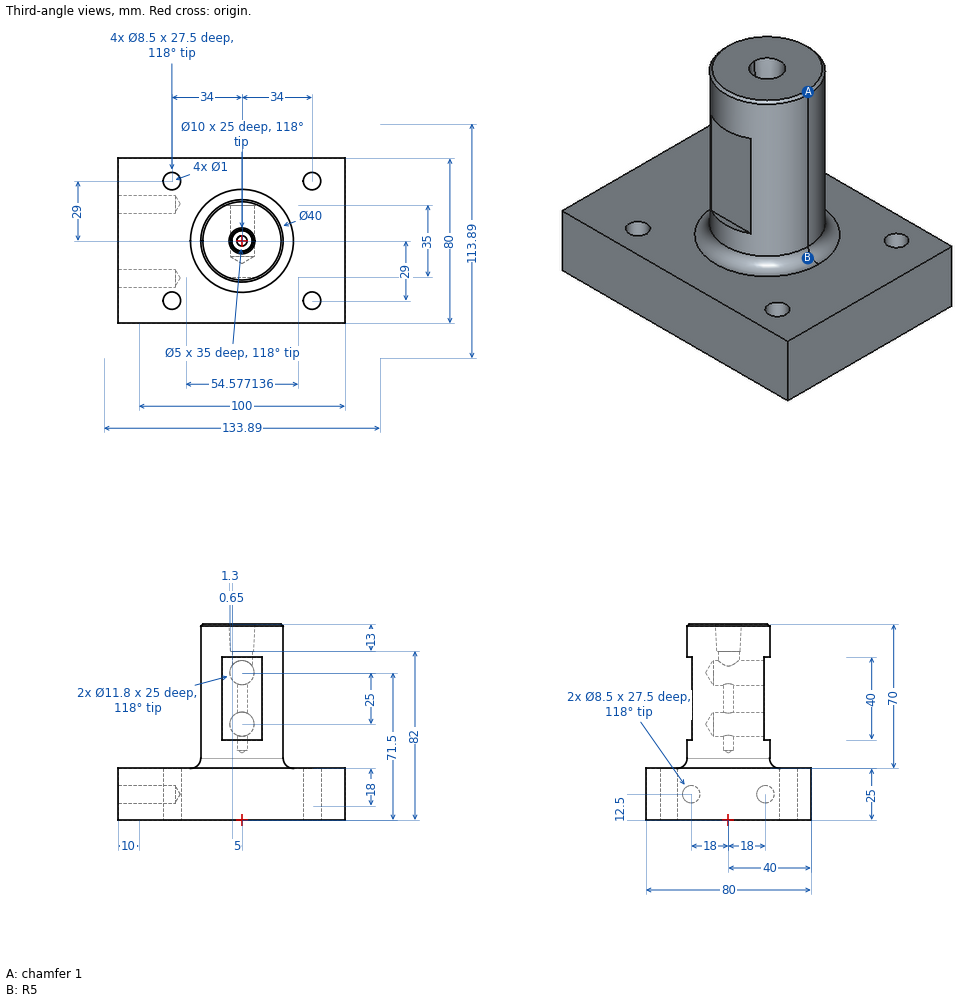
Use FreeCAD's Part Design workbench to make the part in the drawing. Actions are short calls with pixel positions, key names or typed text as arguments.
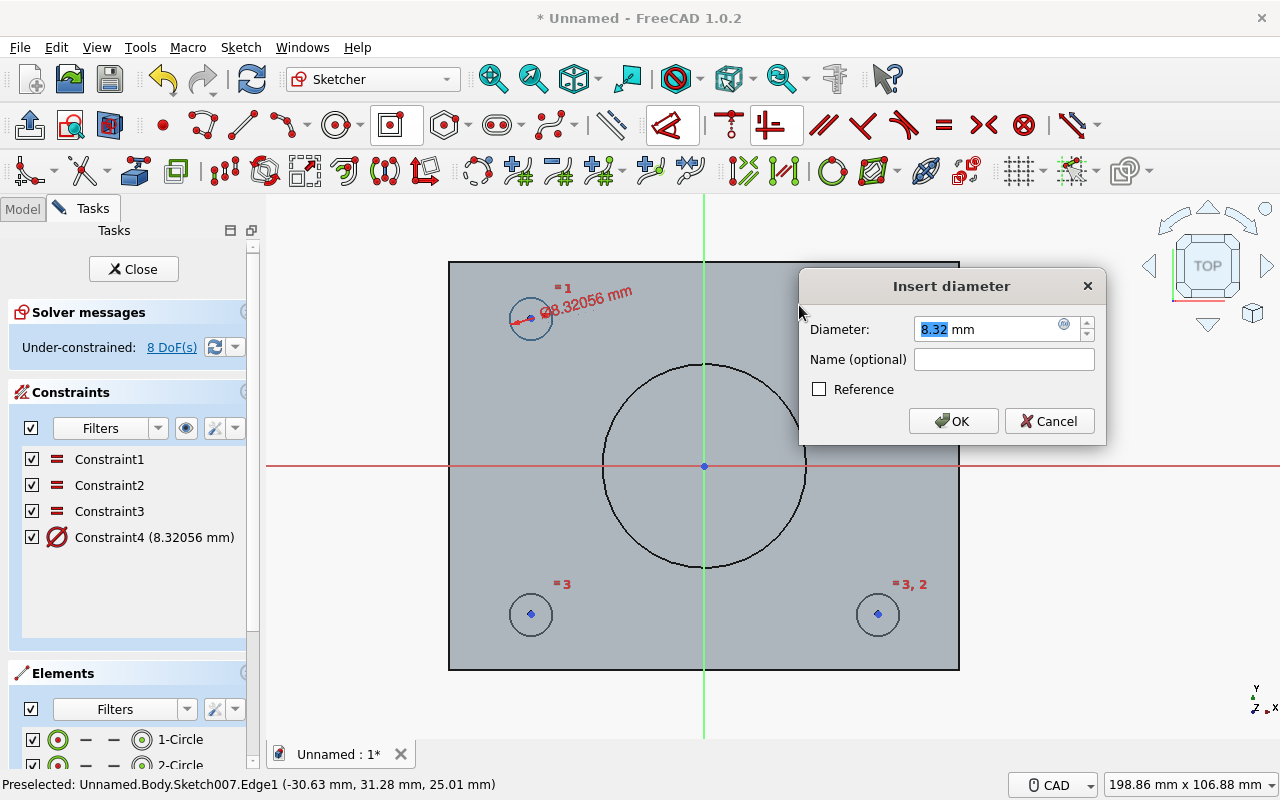
text(8.5)
key(Return)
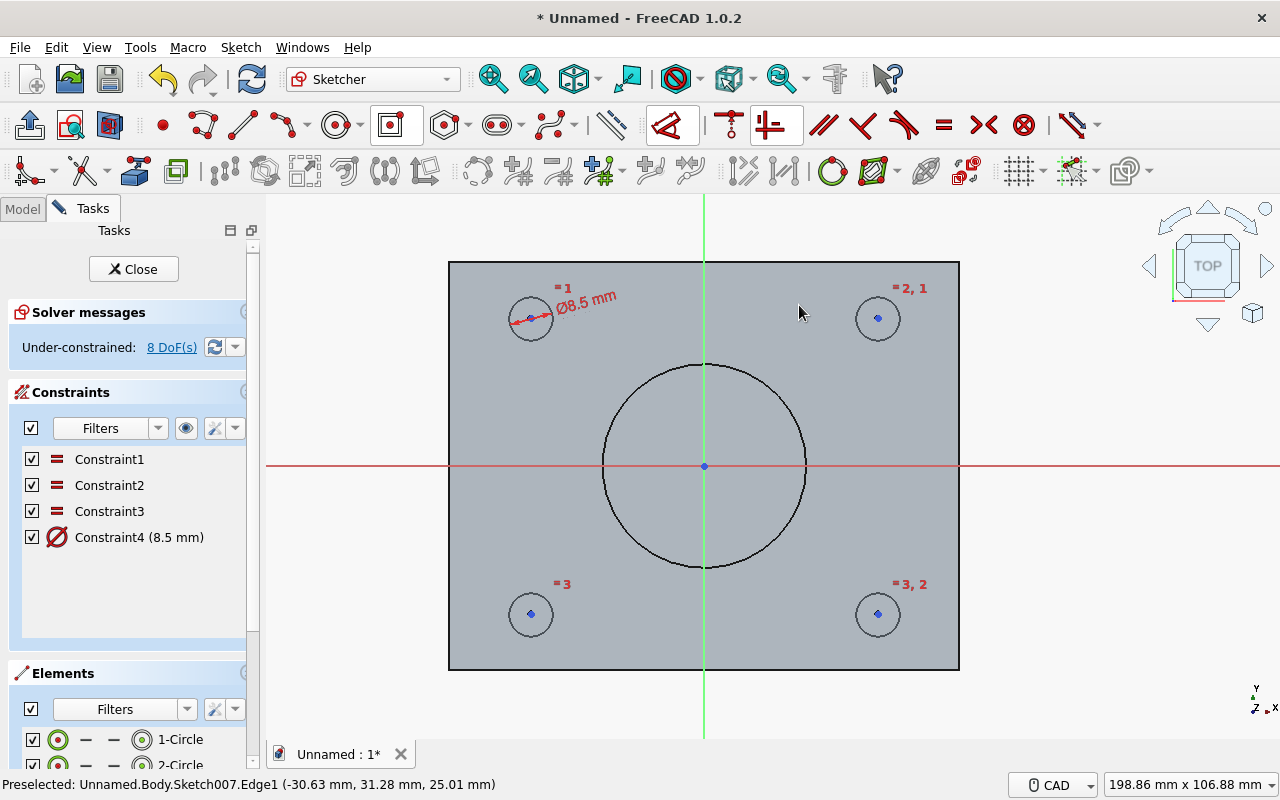
click(531, 319)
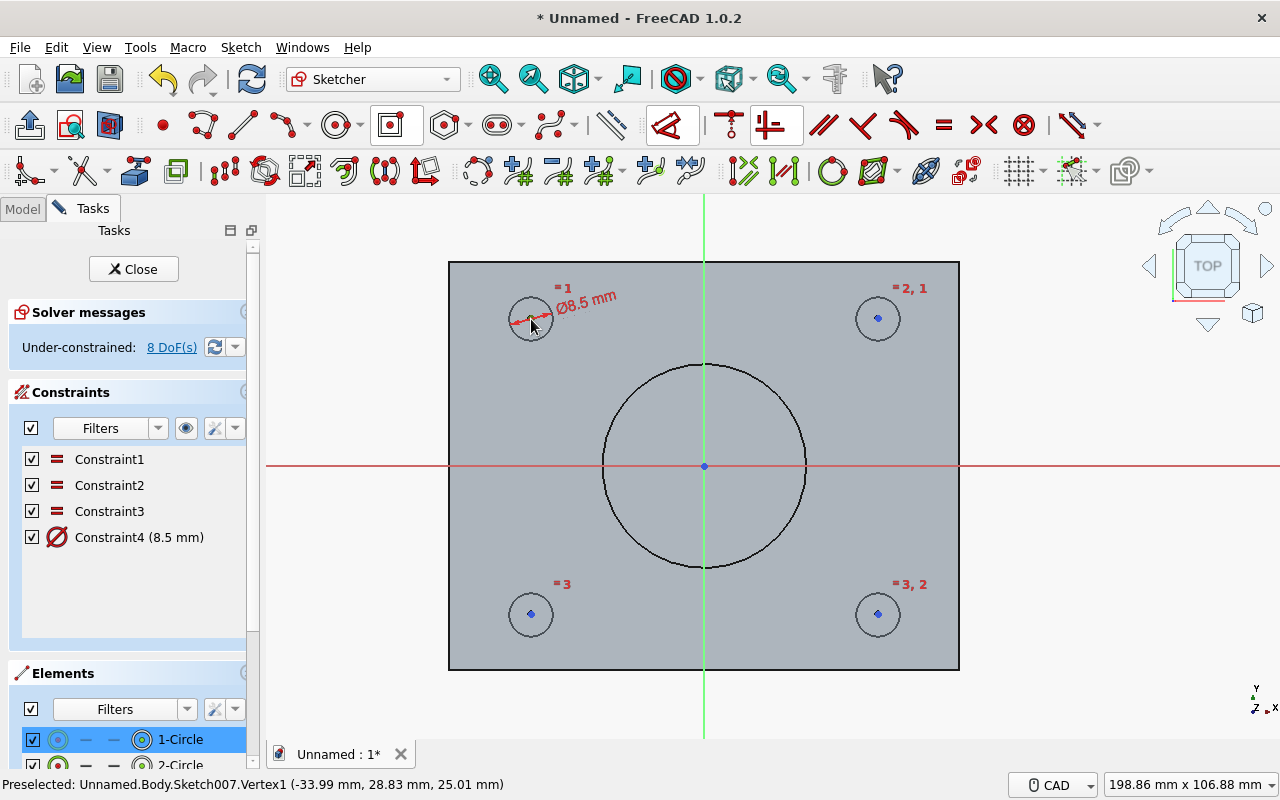
click(694, 126)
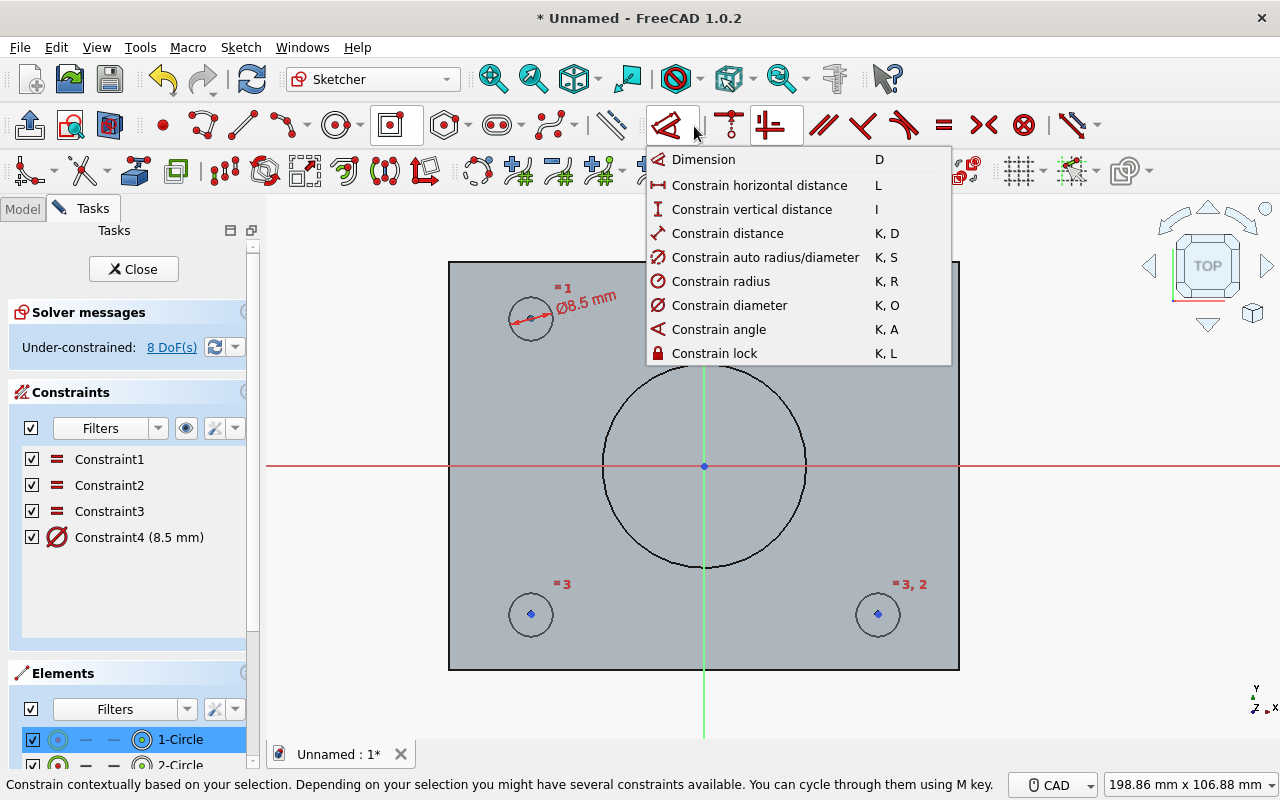
click(799, 185)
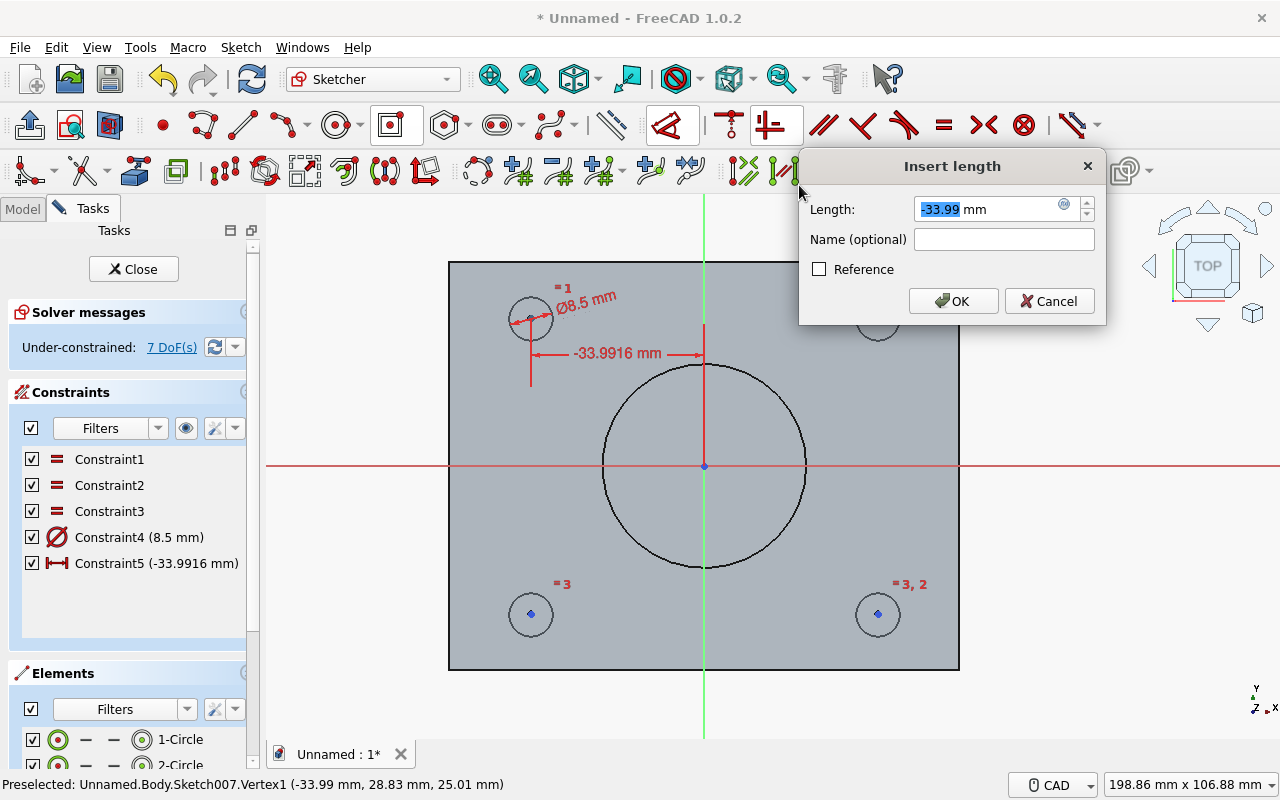
text(-34)
key(Return)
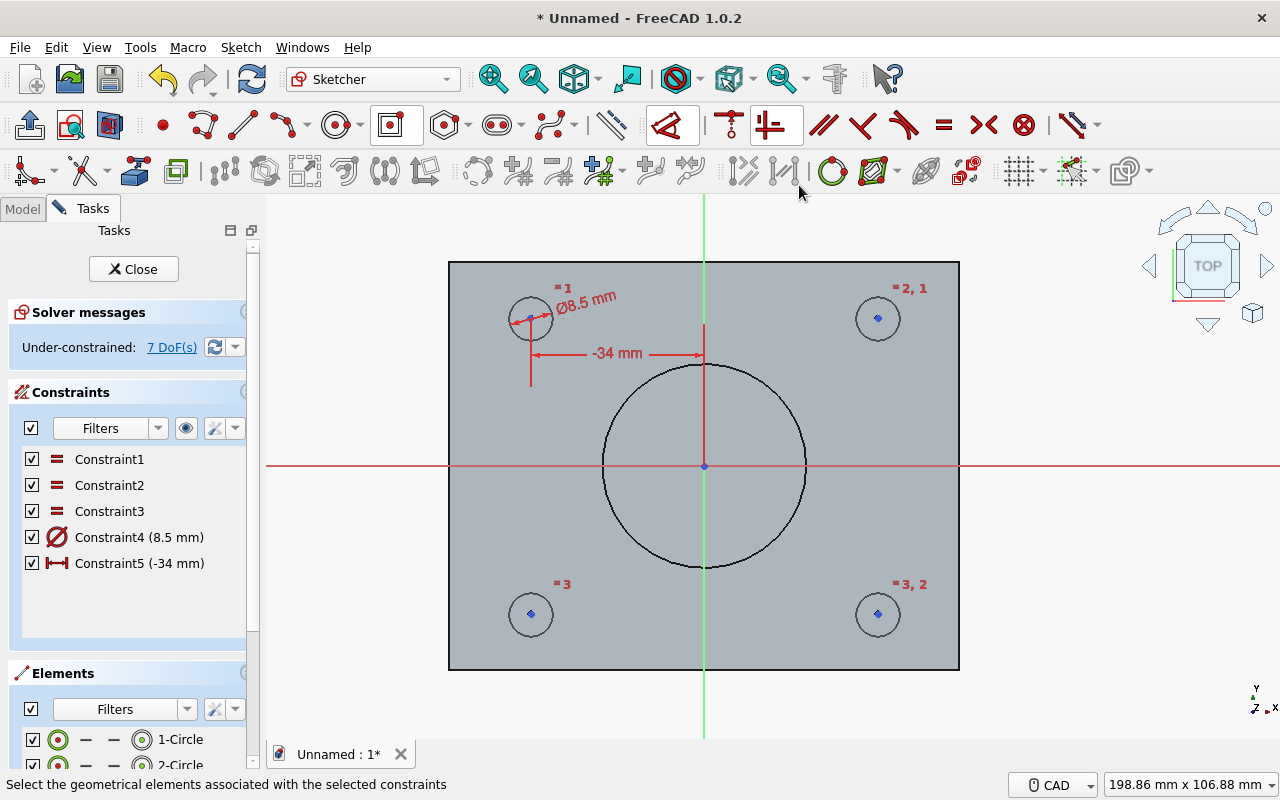
click(531, 319)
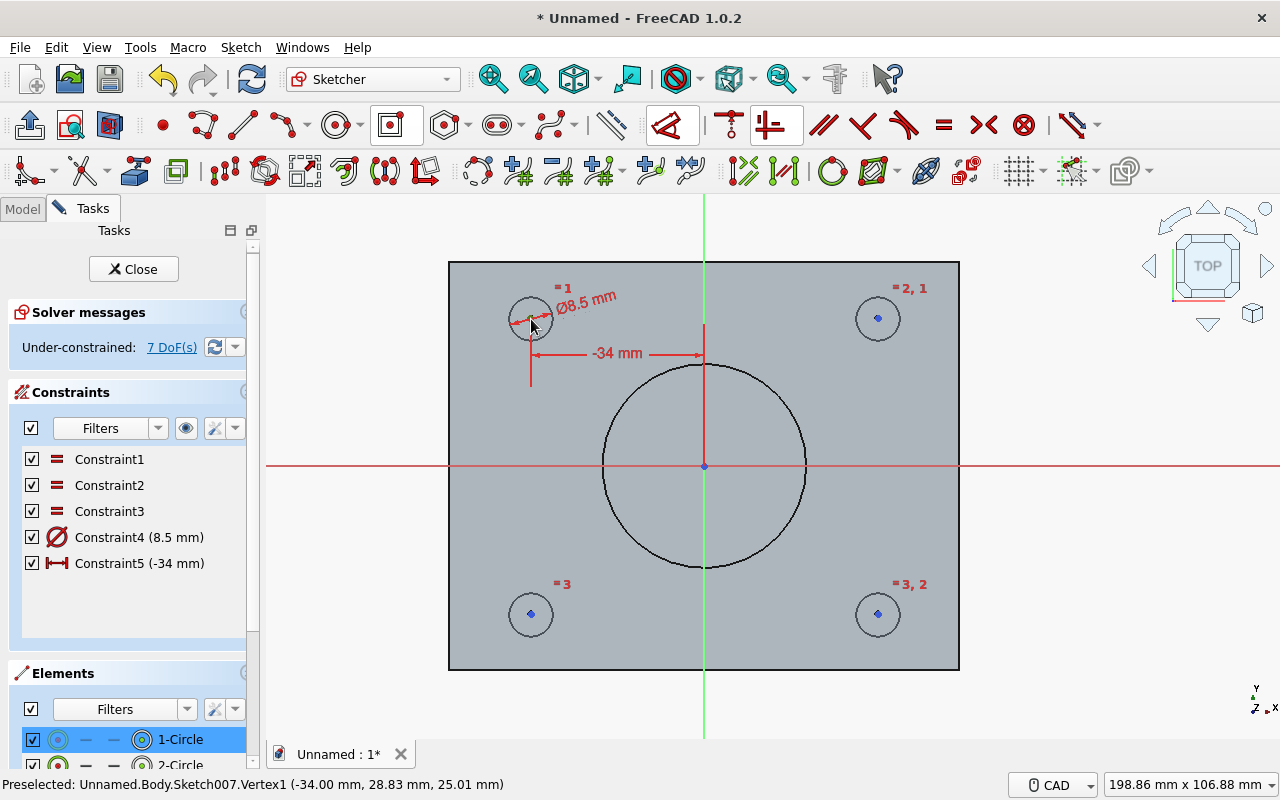
click(694, 126)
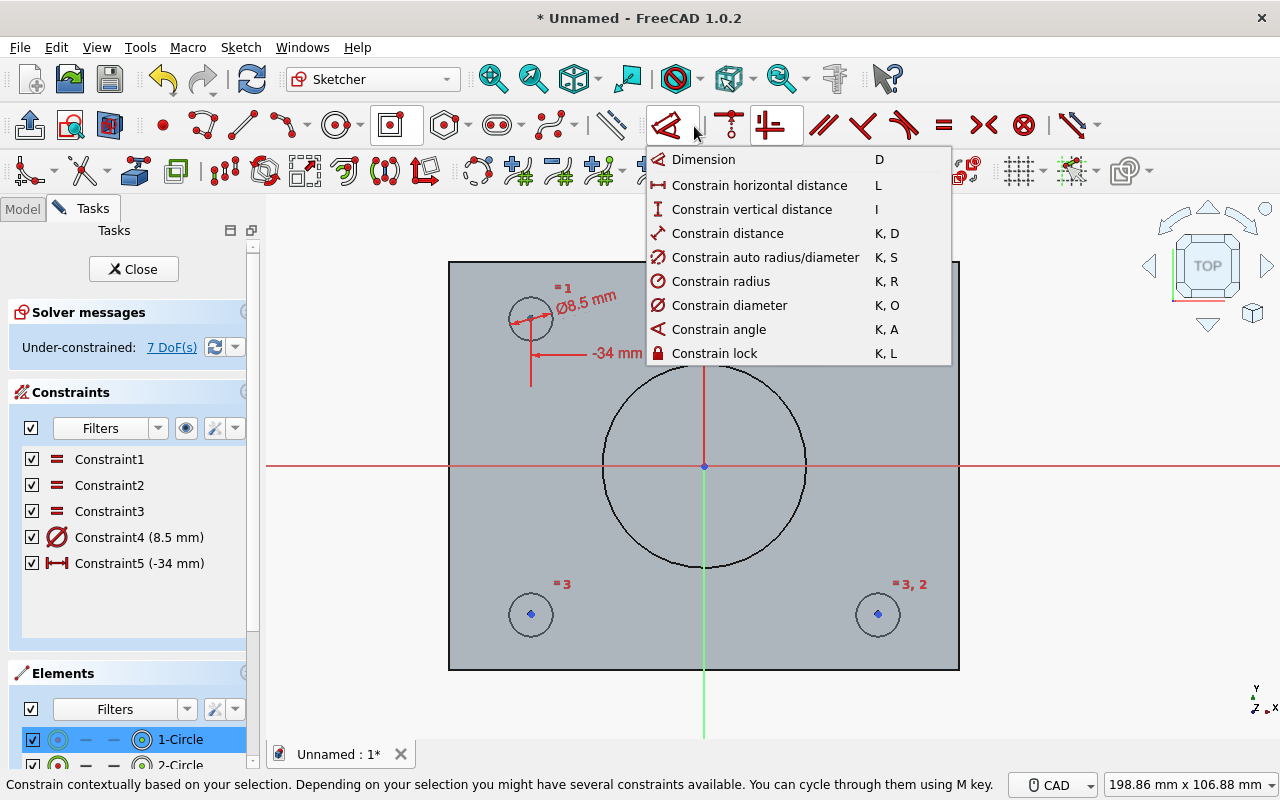
click(799, 209)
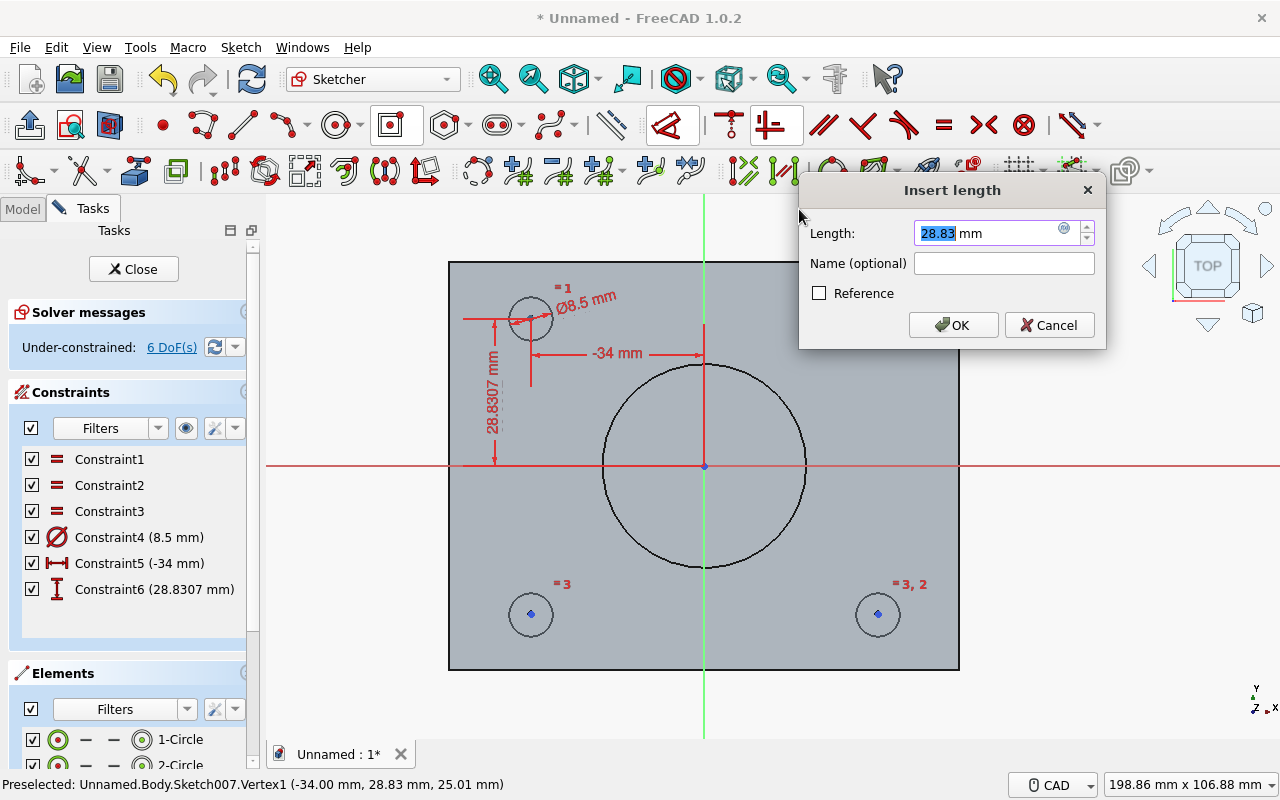
text(29)
key(Return)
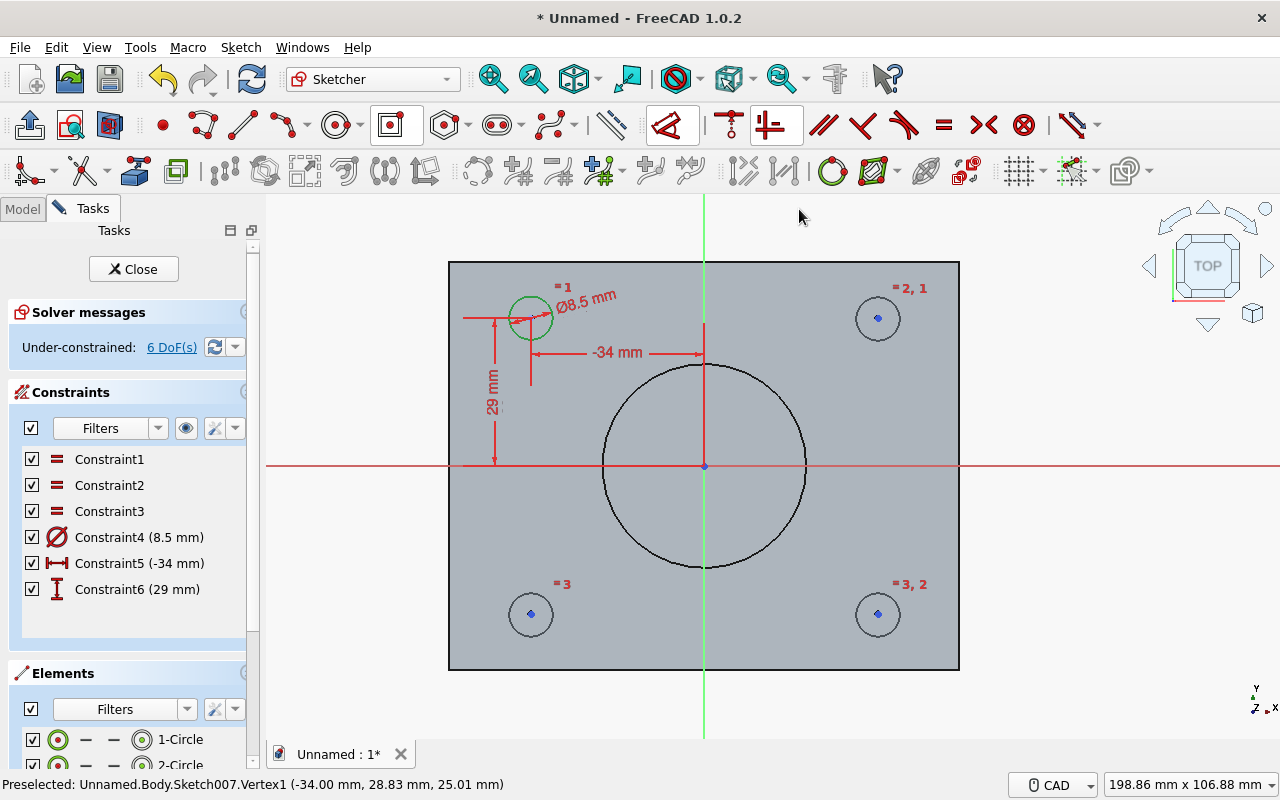
click(878, 319)